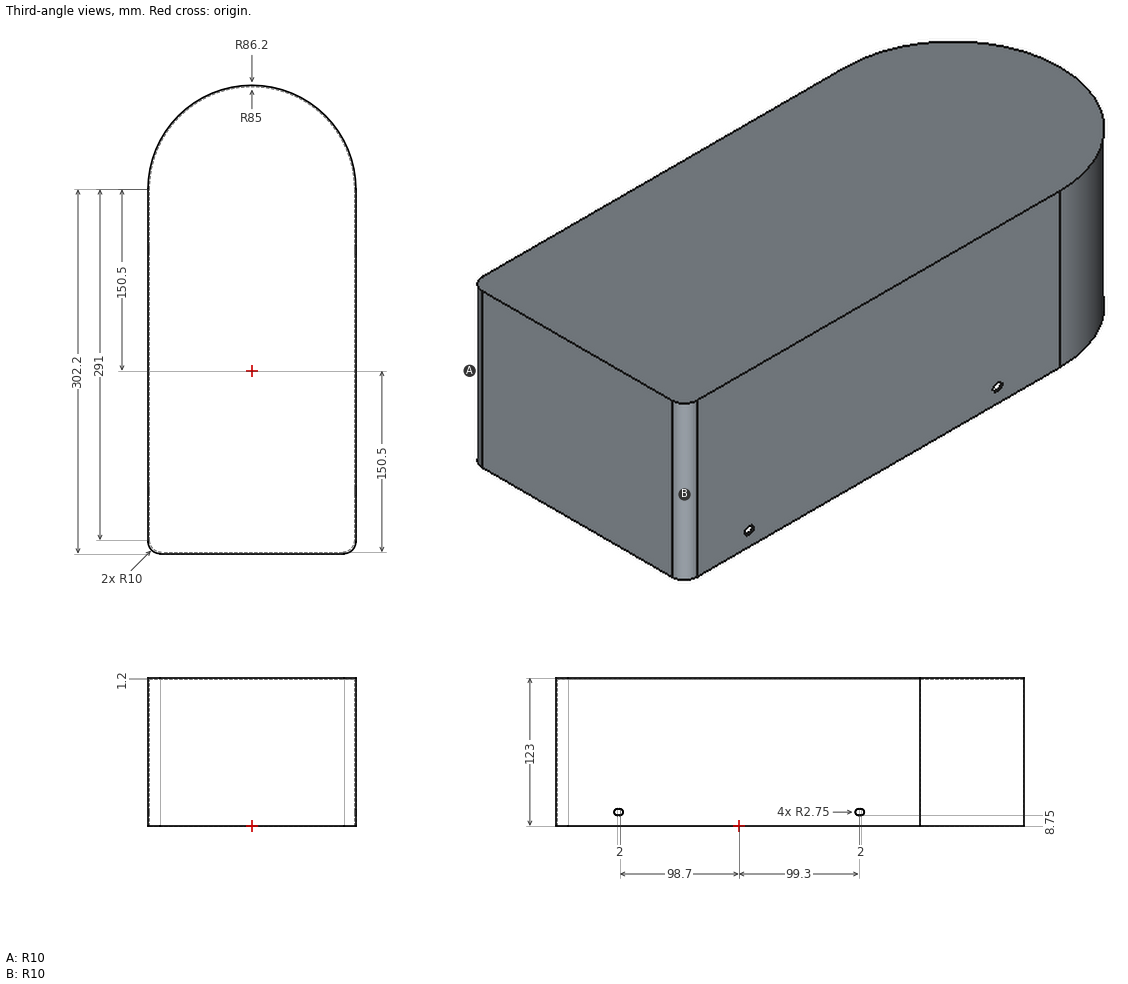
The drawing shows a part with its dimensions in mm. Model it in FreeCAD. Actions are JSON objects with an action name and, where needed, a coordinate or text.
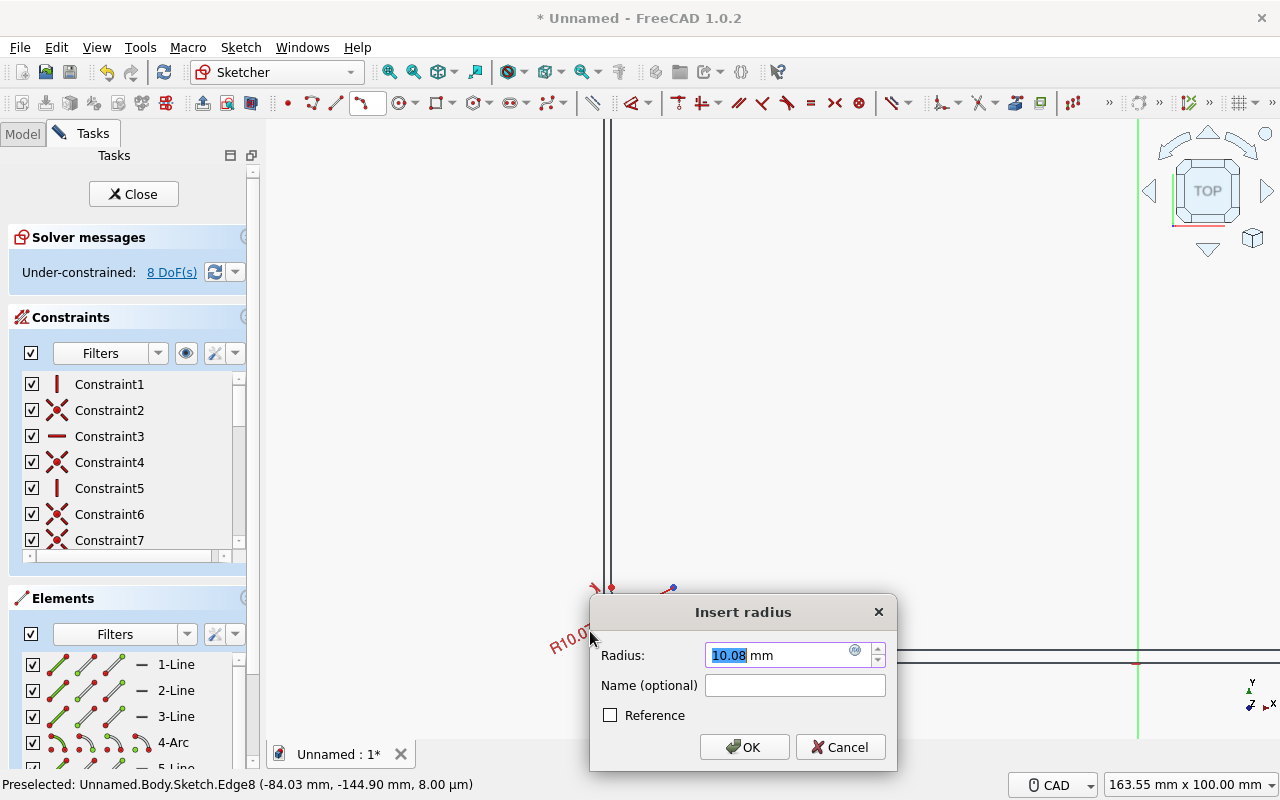
{"action": "type", "text": "10"}
{"action": "key", "text": "Return"}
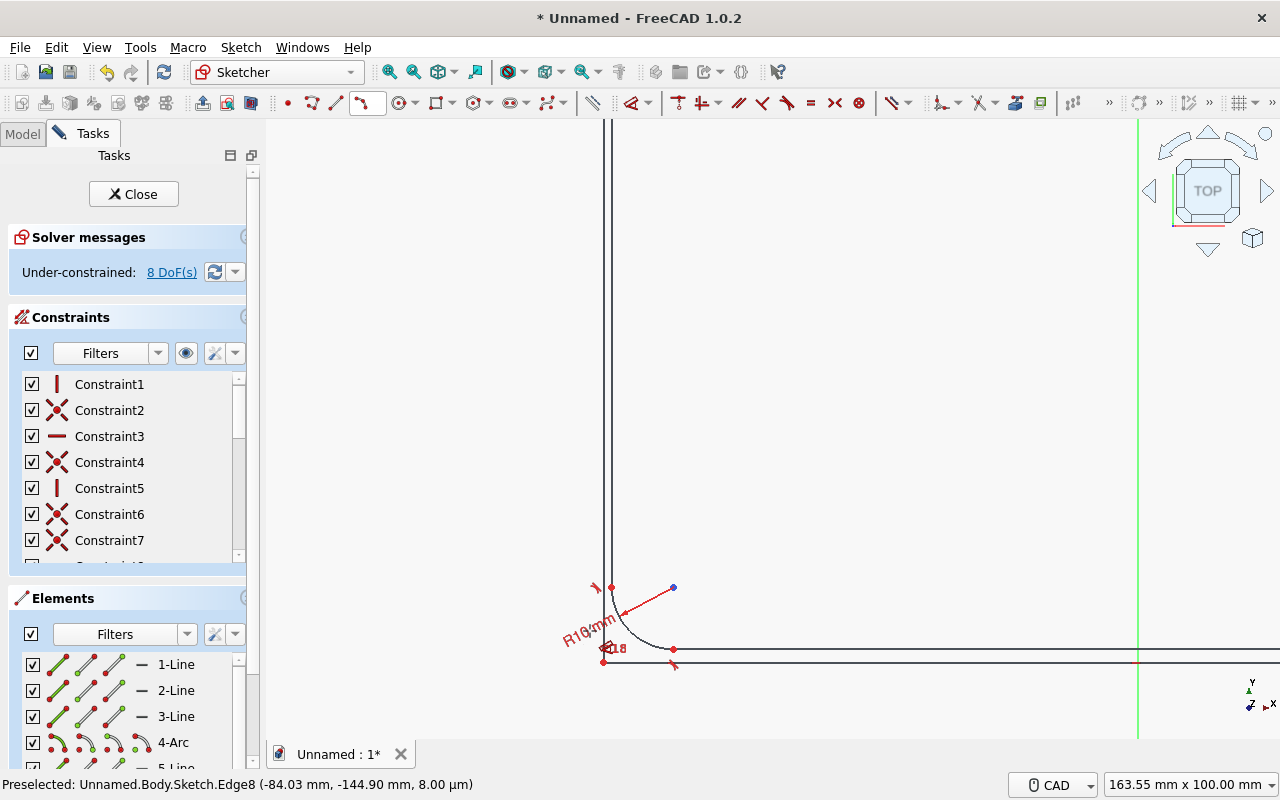
{"action": "scroll", "coordinate": [619, 622], "scroll_direction": "down", "scroll_amount": 9}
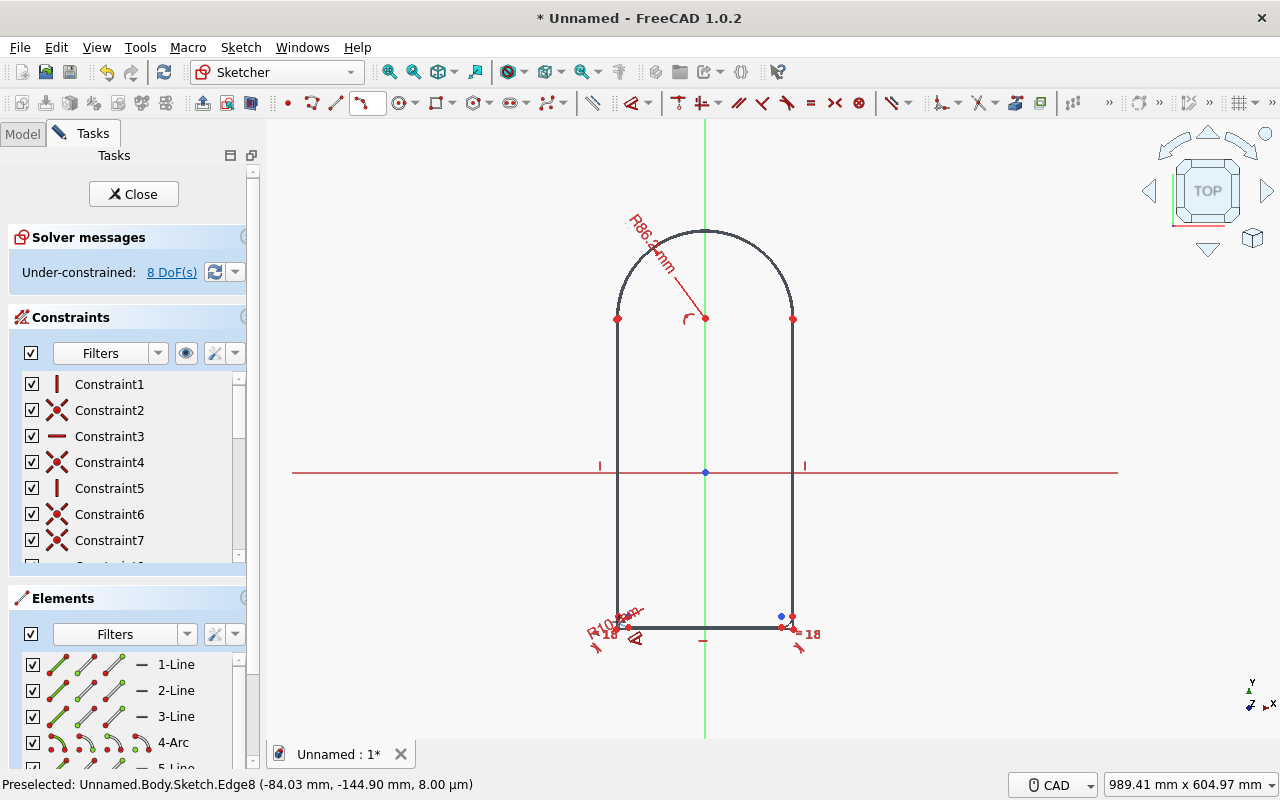
{"action": "scroll", "coordinate": [756, 248], "scroll_direction": "up", "scroll_amount": 12}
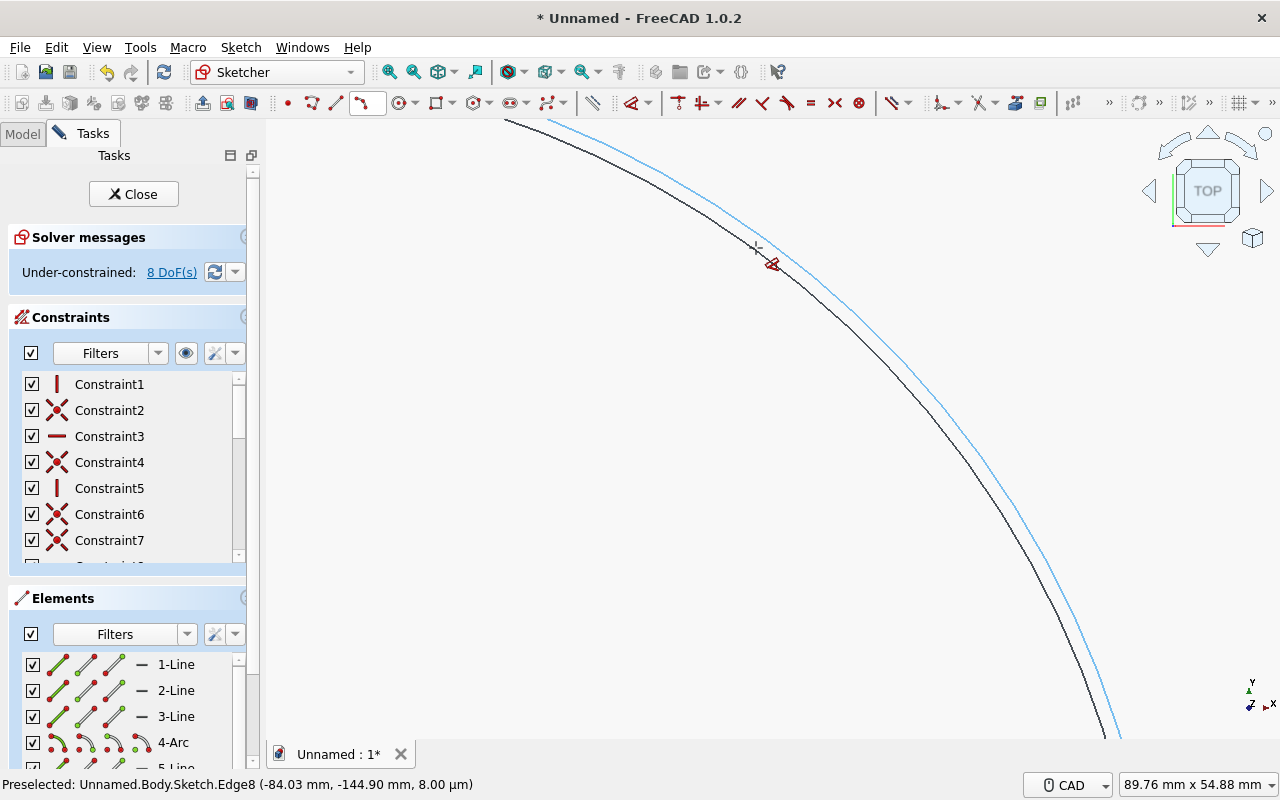
{"action": "left_click", "coordinate": [754, 249]}
{"action": "left_click", "coordinate": [773, 223]}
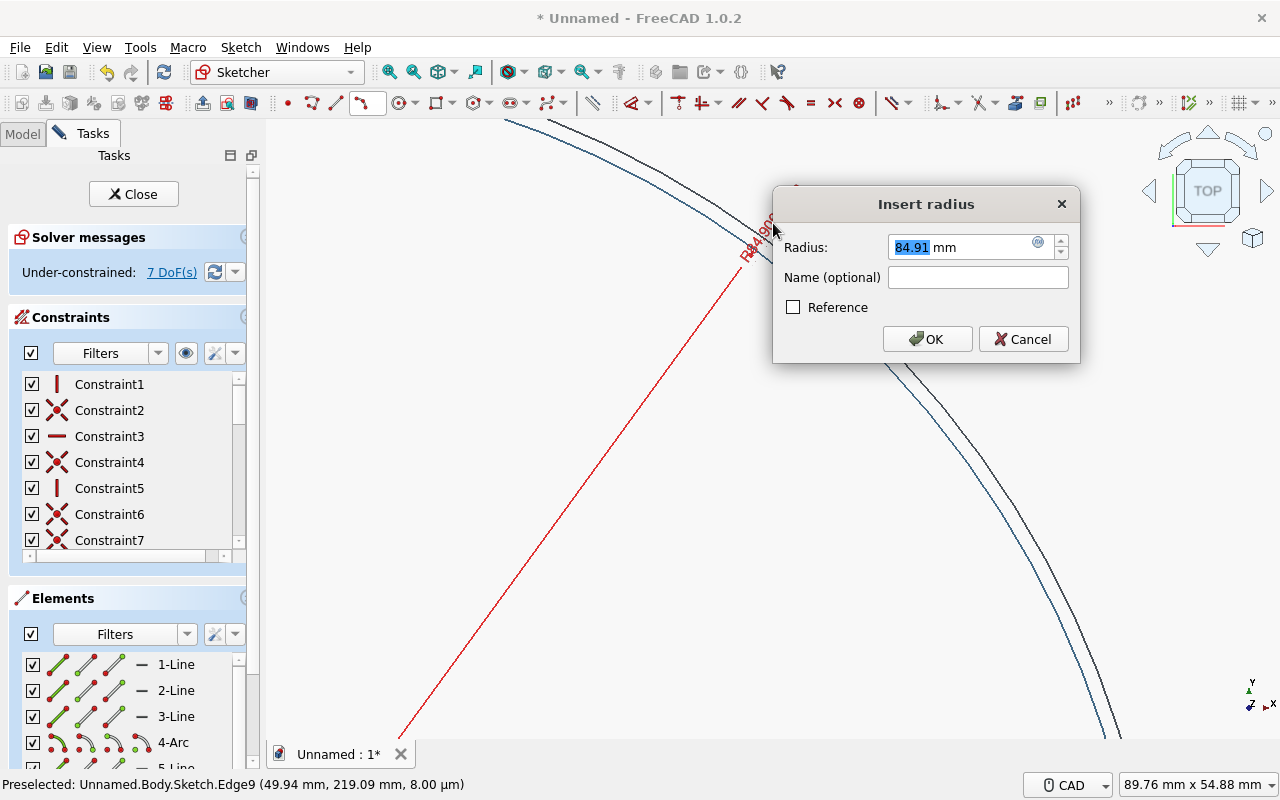
{"action": "type", "text": "85"}
{"action": "key", "text": "Return"}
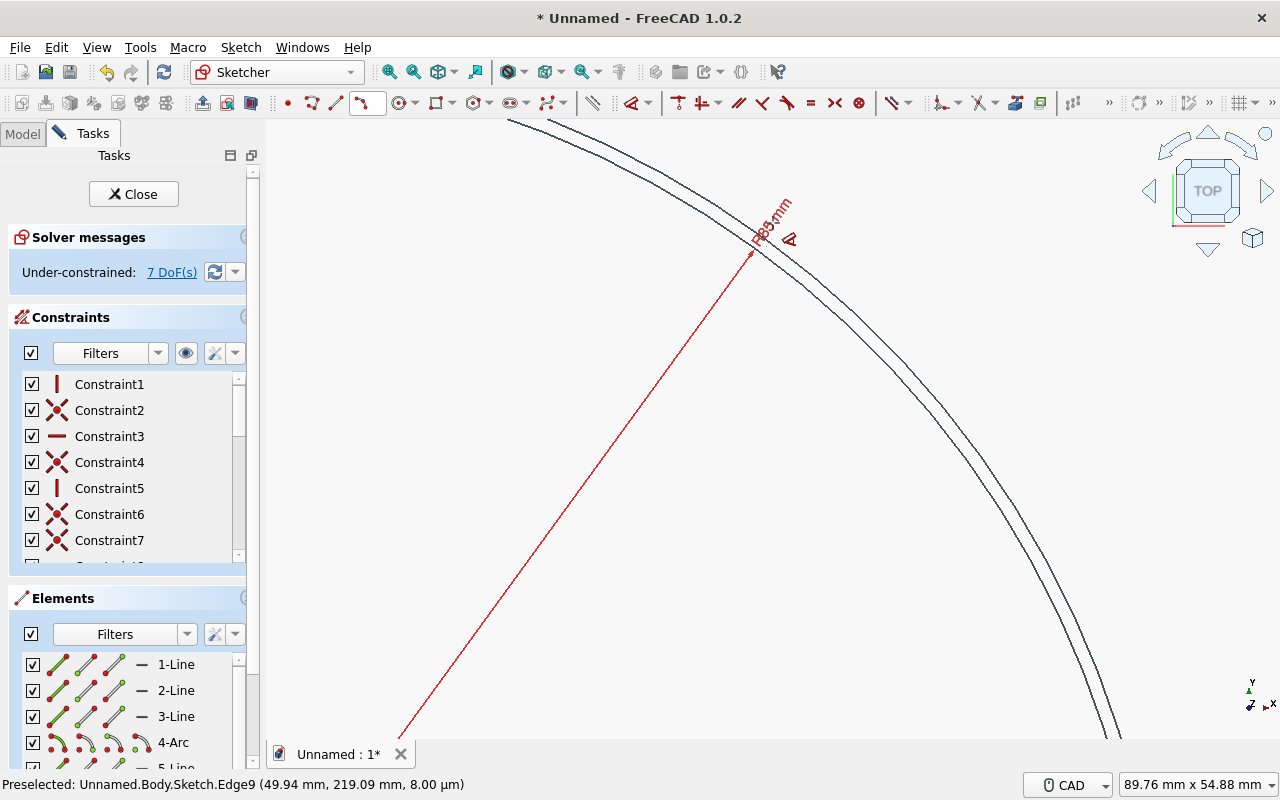
{"action": "scroll", "coordinate": [756, 248], "scroll_direction": "down", "scroll_amount": 12}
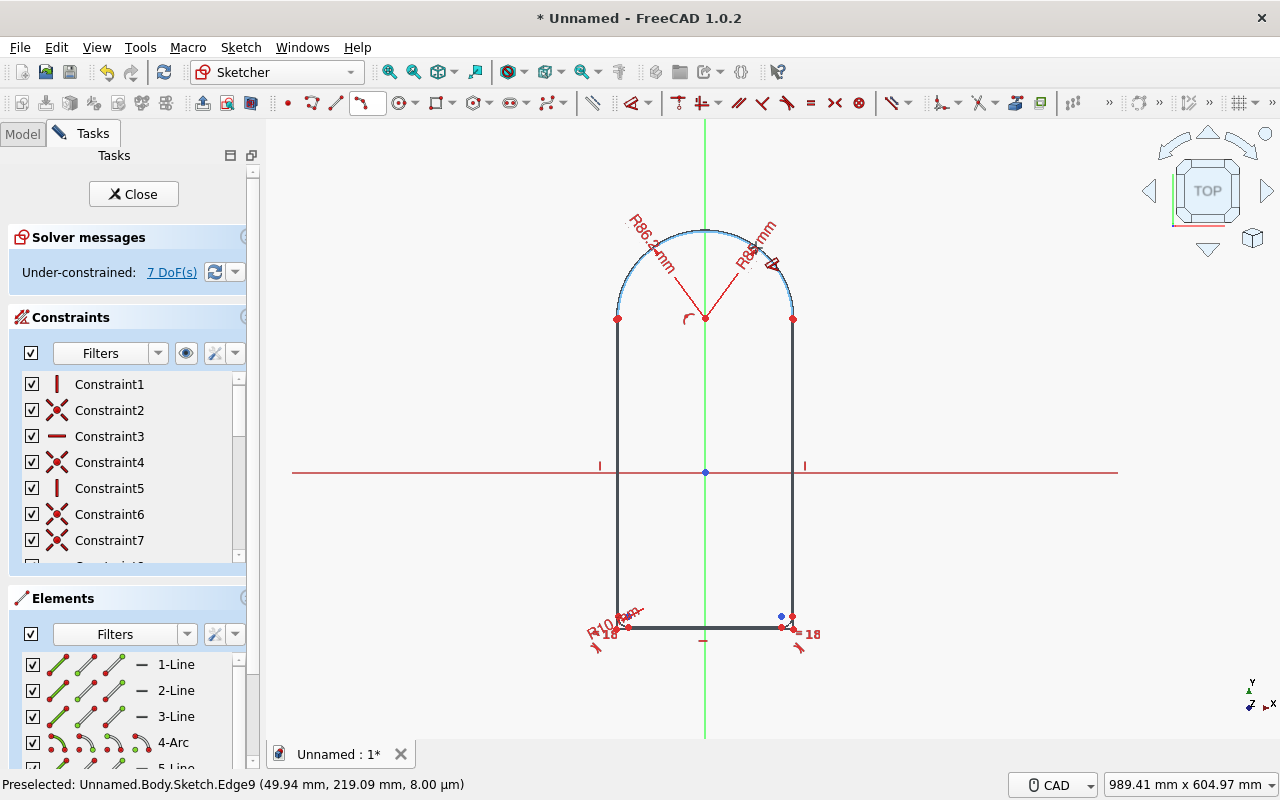
{"action": "scroll", "coordinate": [618, 527], "scroll_direction": "up", "scroll_amount": 13}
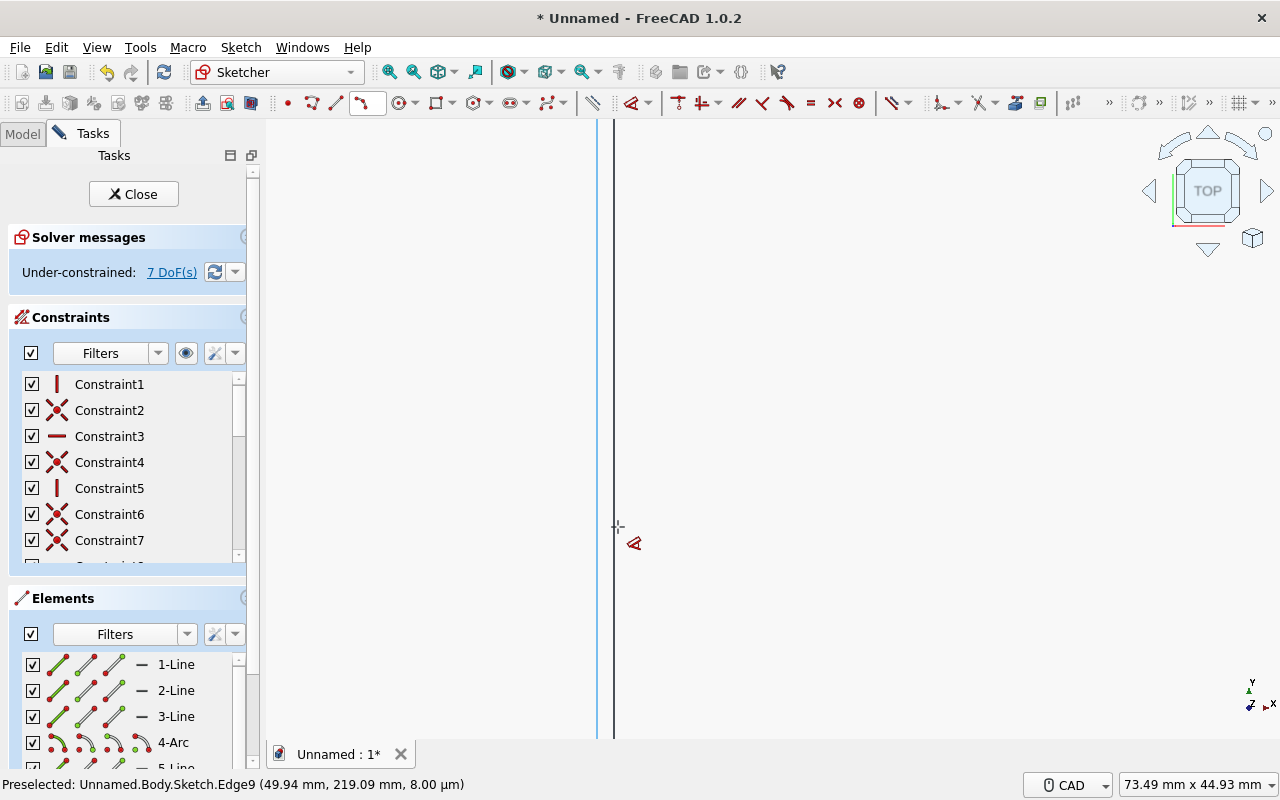
{"action": "left_click", "coordinate": [614, 525]}
{"action": "left_click", "coordinate": [580, 429]}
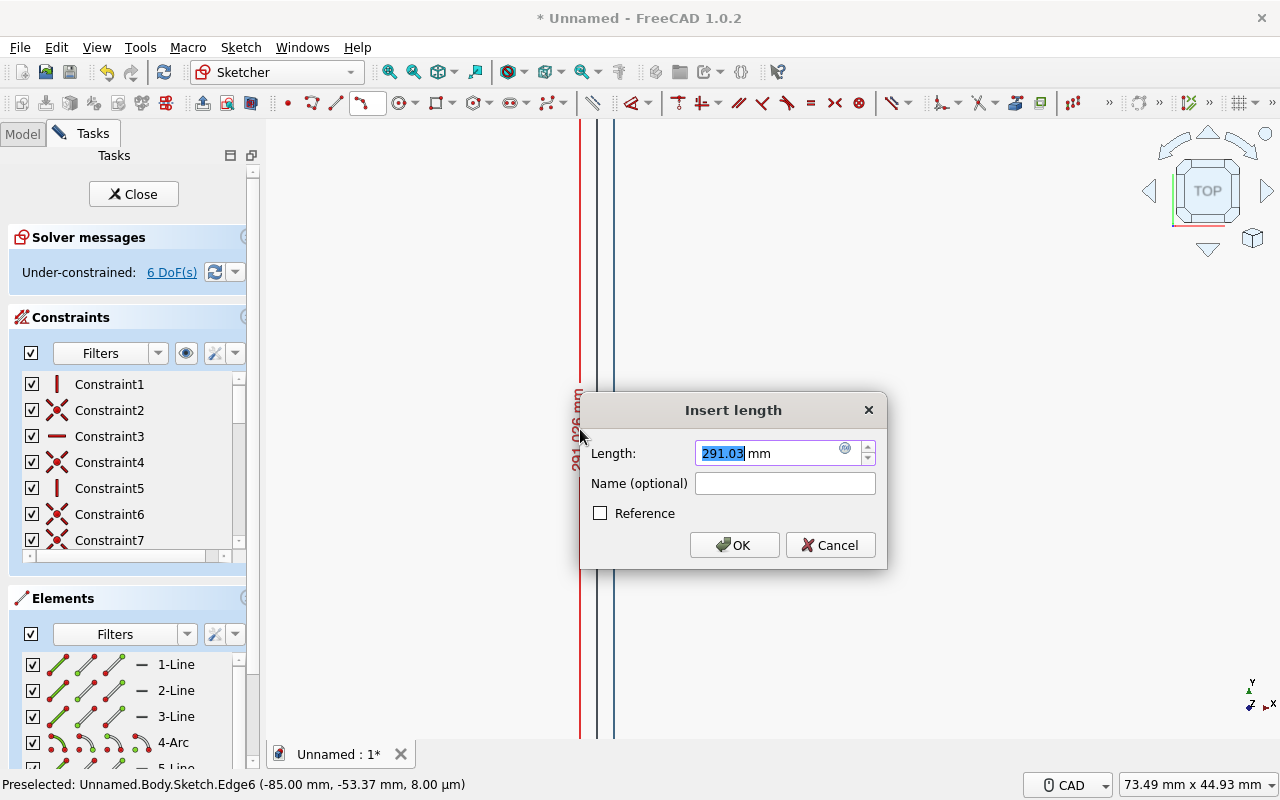
{"action": "type", "text": "291"}
{"action": "key", "text": "Return"}